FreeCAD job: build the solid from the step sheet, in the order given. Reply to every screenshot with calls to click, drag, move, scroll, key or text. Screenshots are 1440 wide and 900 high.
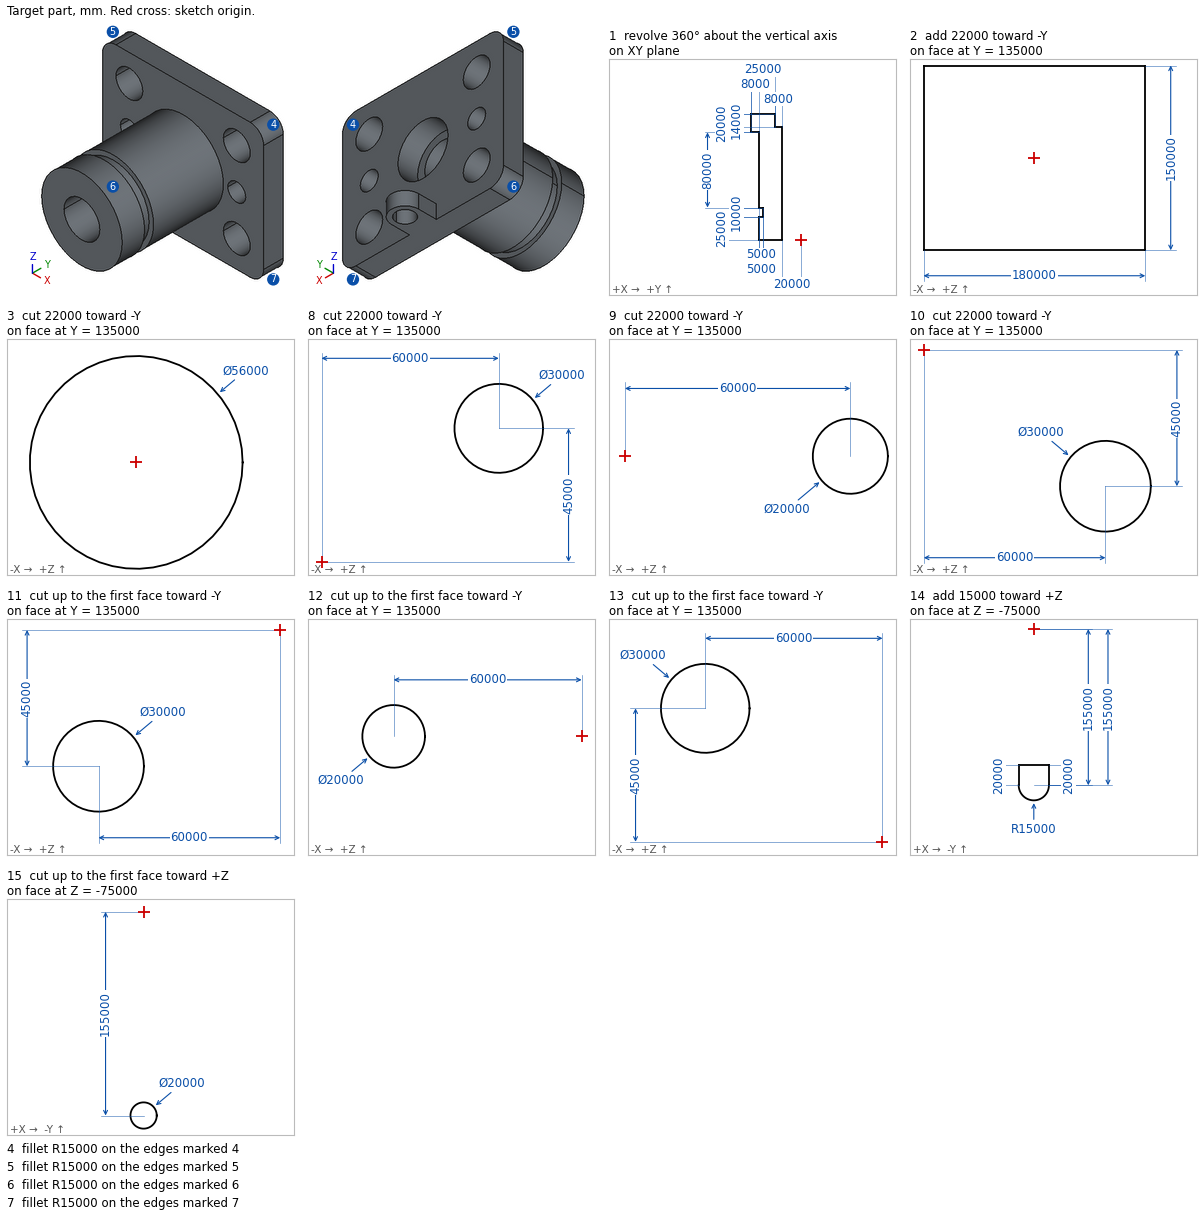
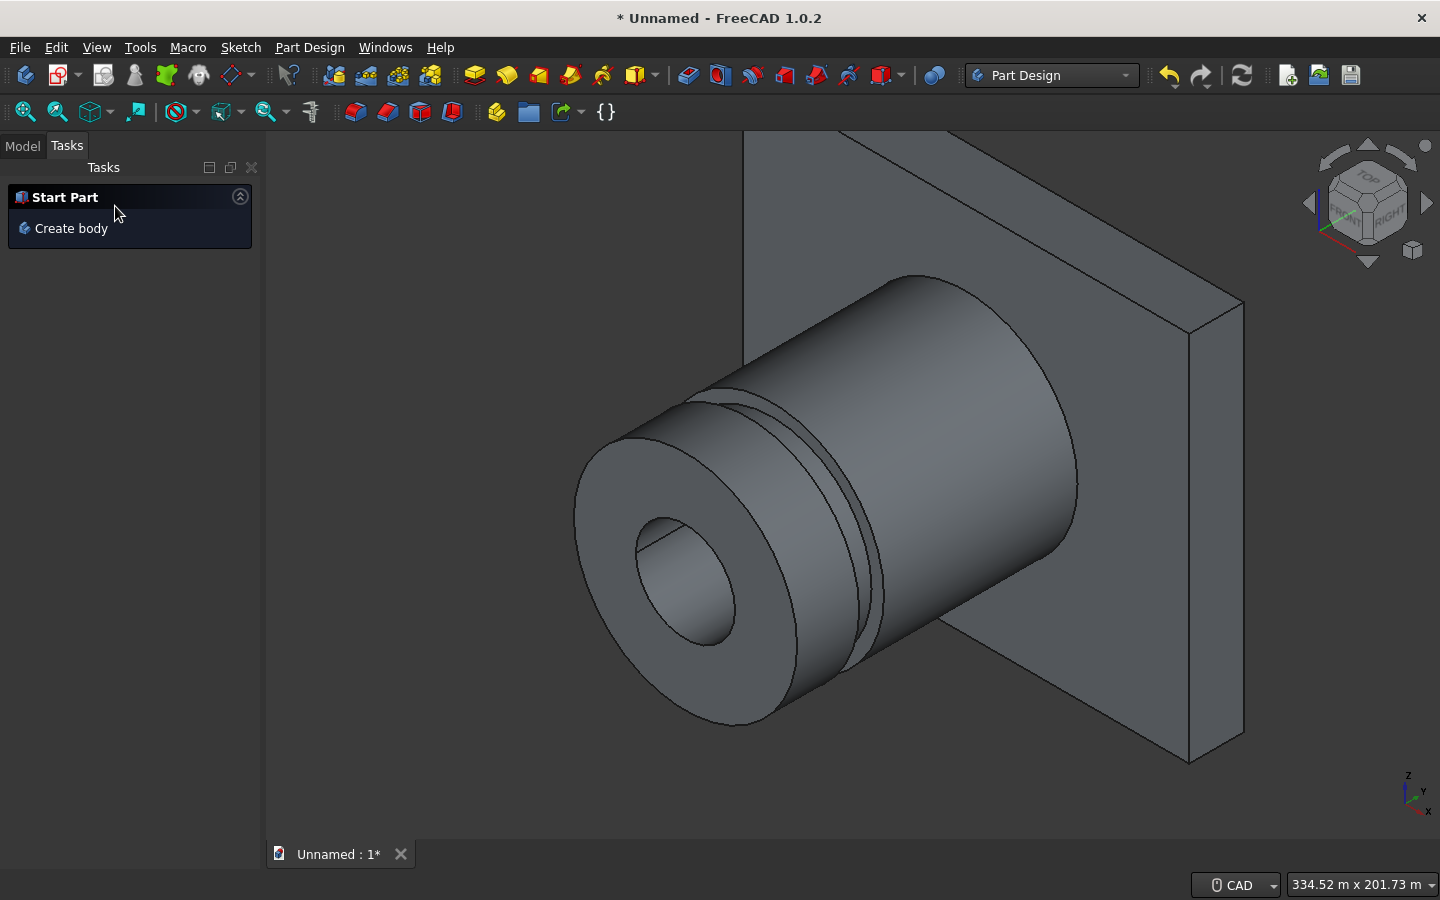
click(26, 112)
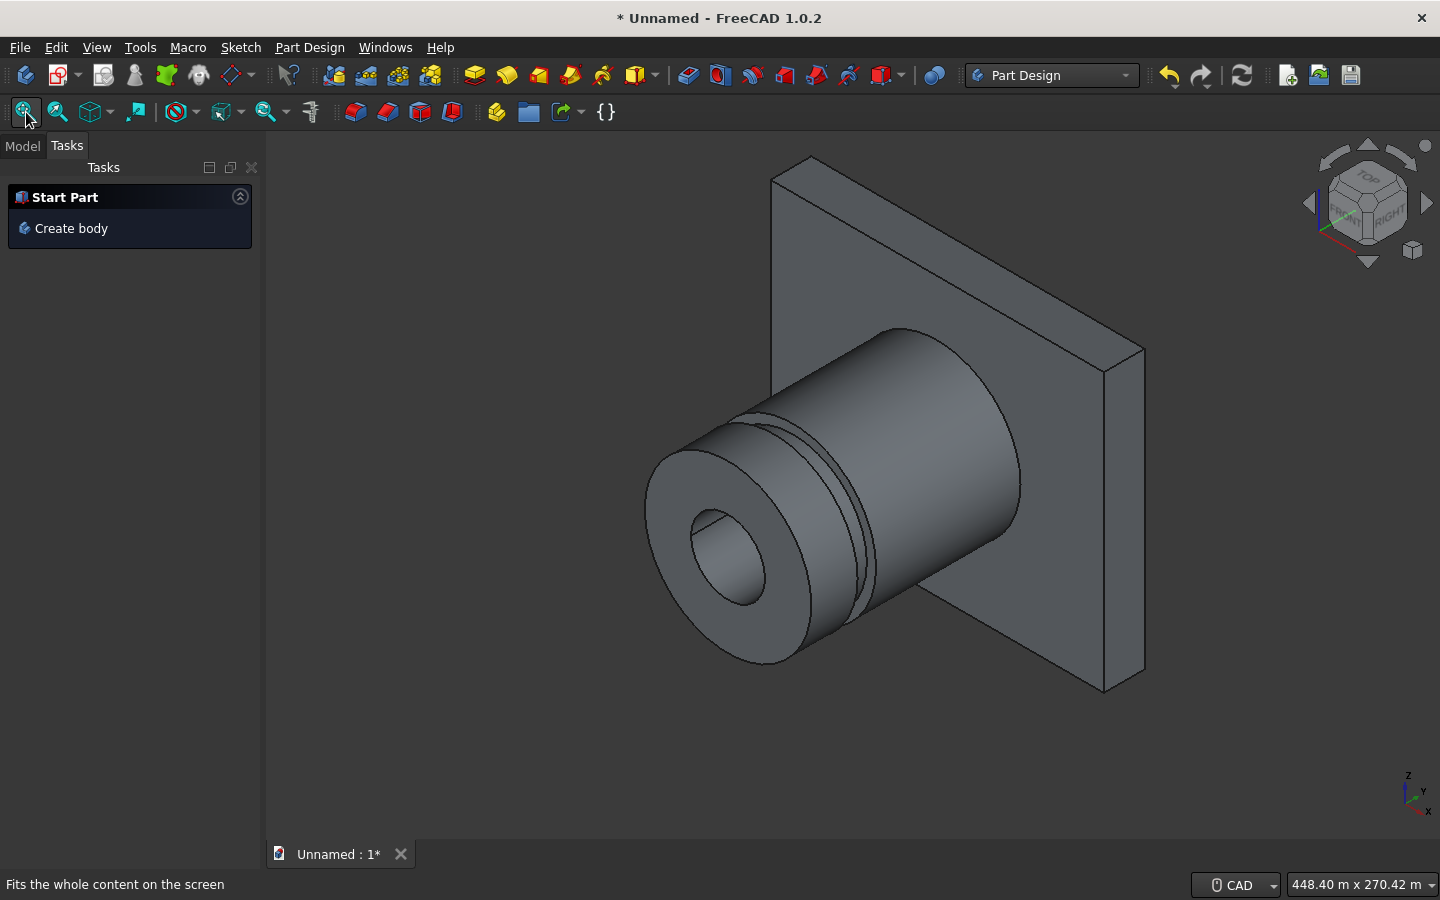
click(1124, 359)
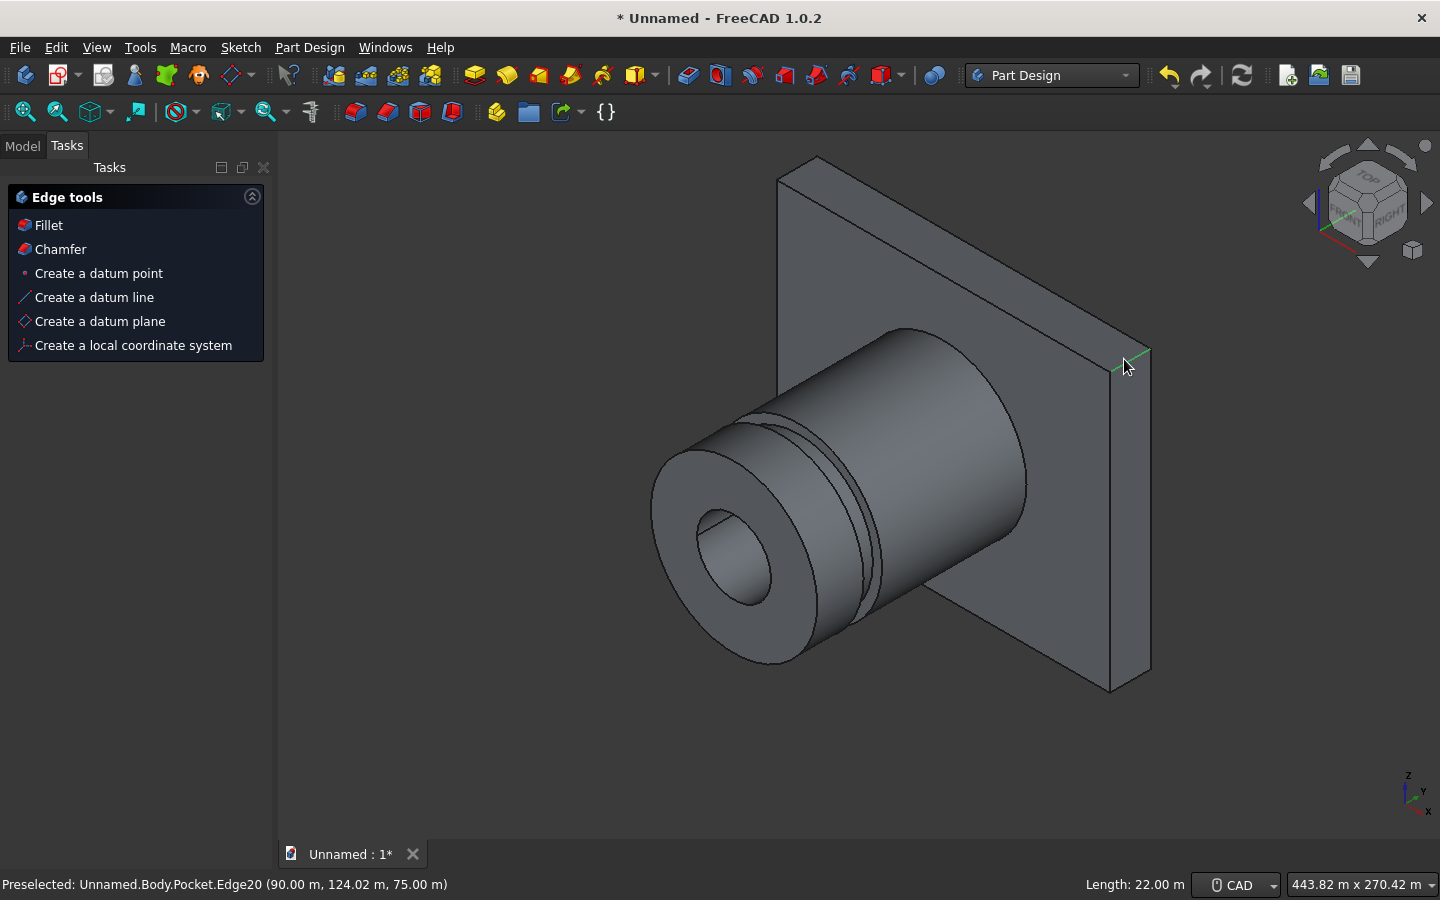
click(356, 112)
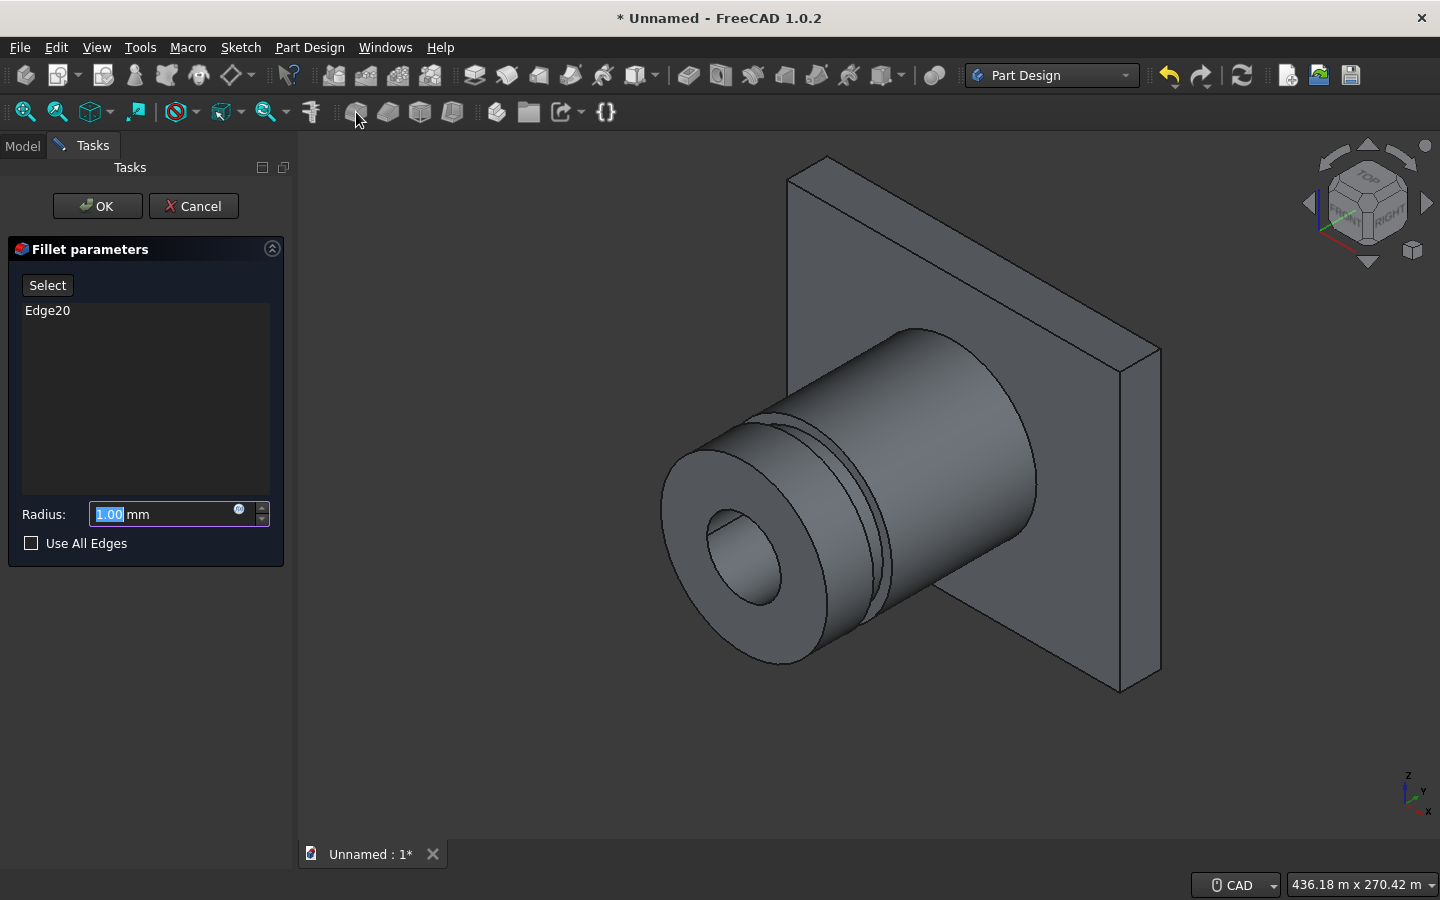
text(15000)
key(Tab)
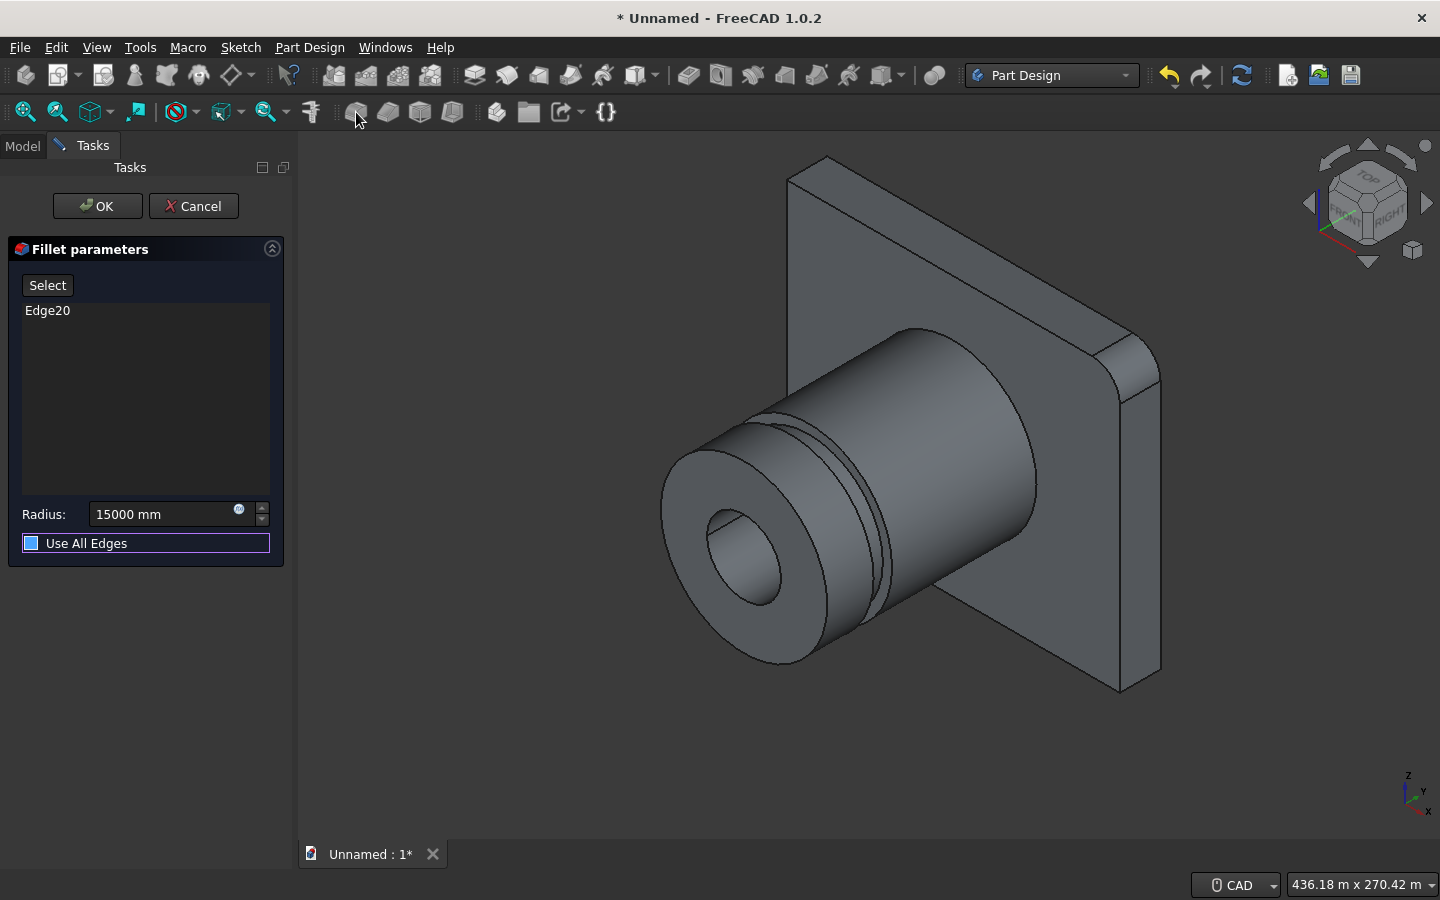
click(98, 206)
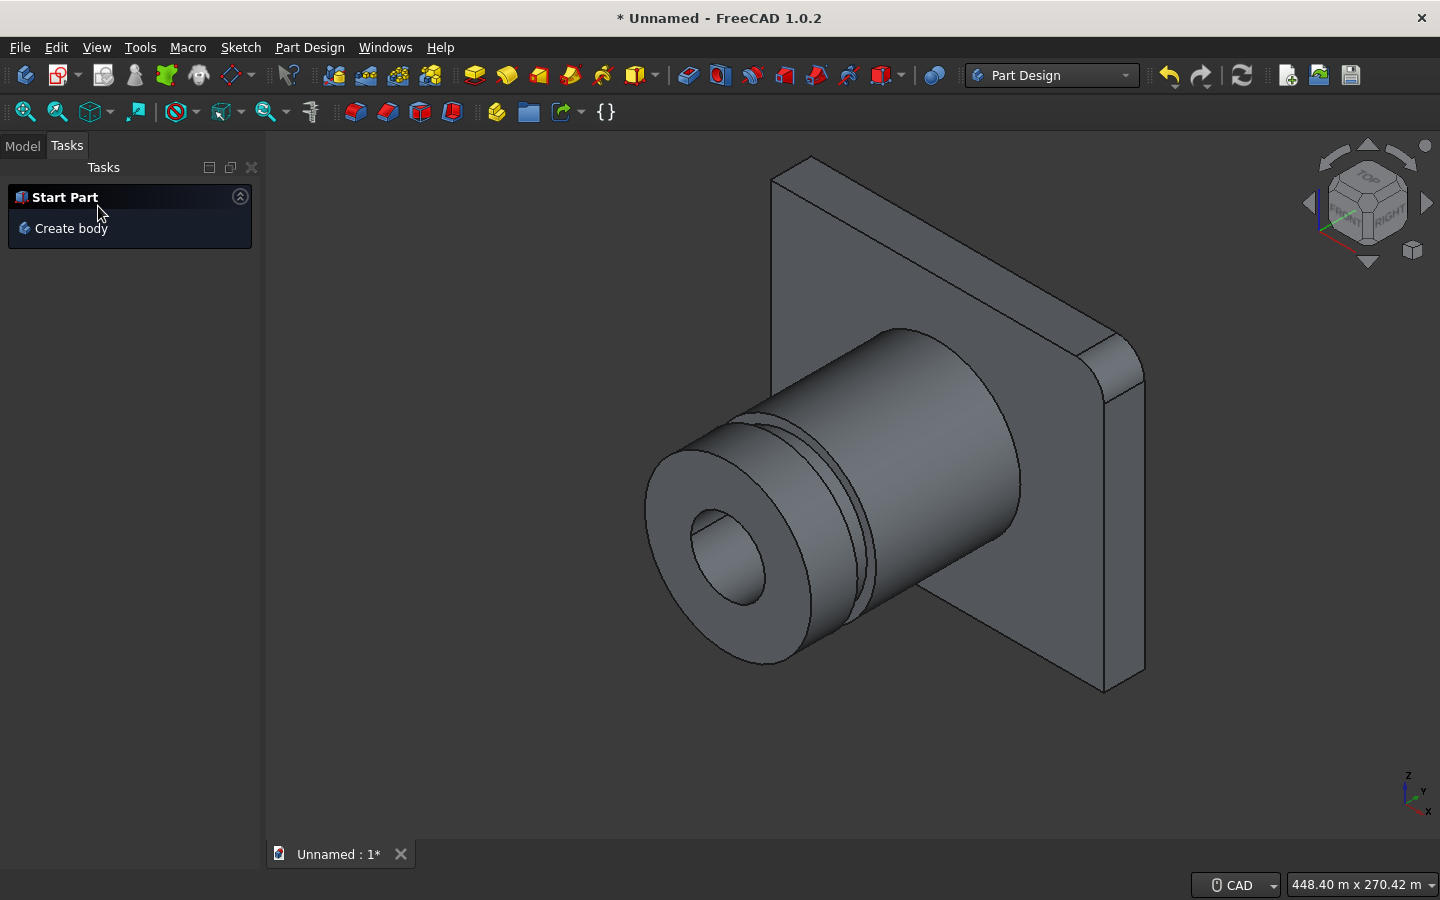
key(2)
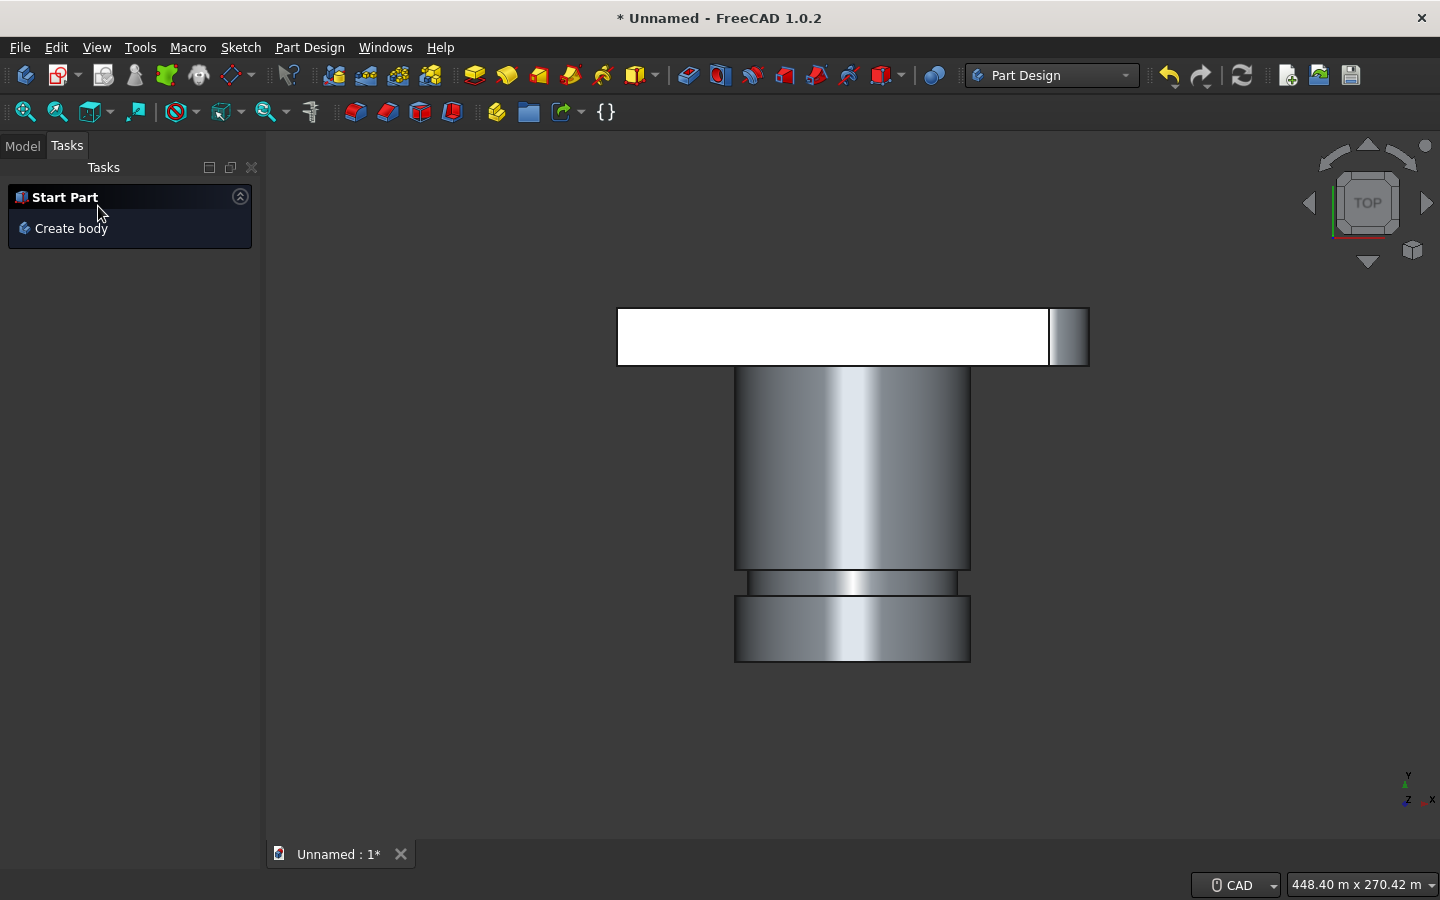
click(617, 336)